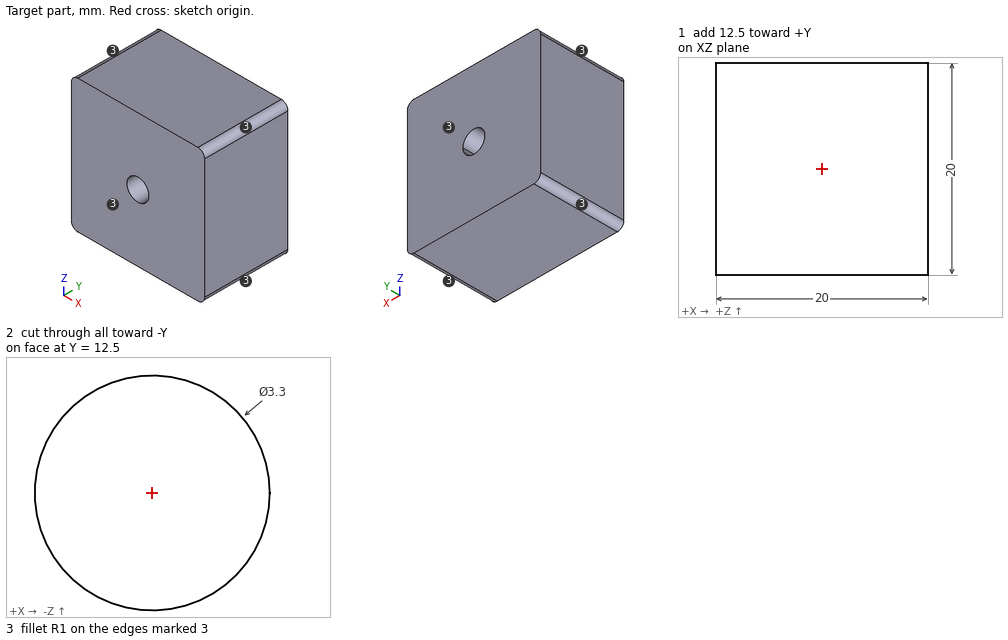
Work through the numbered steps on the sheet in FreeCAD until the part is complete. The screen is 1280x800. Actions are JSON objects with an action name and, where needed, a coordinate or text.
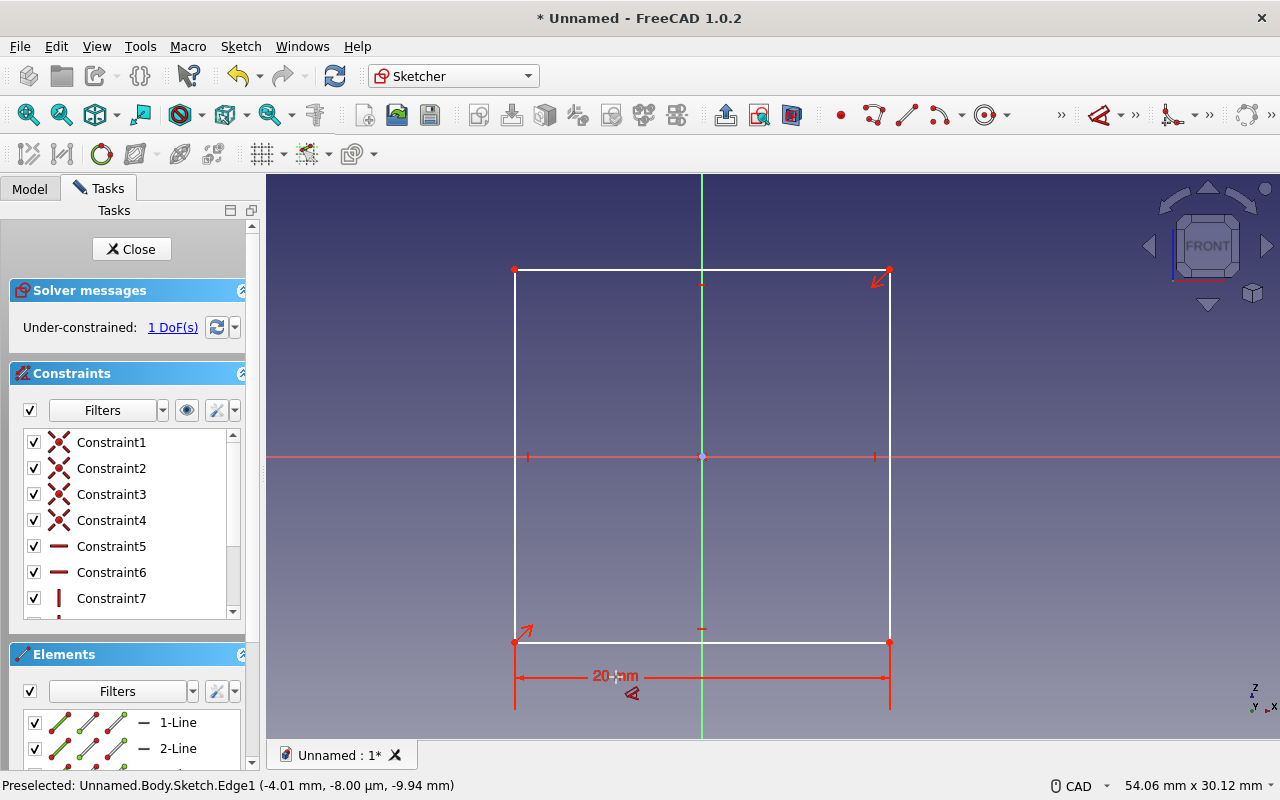
{"action": "left_click", "coordinate": [890, 531]}
{"action": "left_click", "coordinate": [924, 371]}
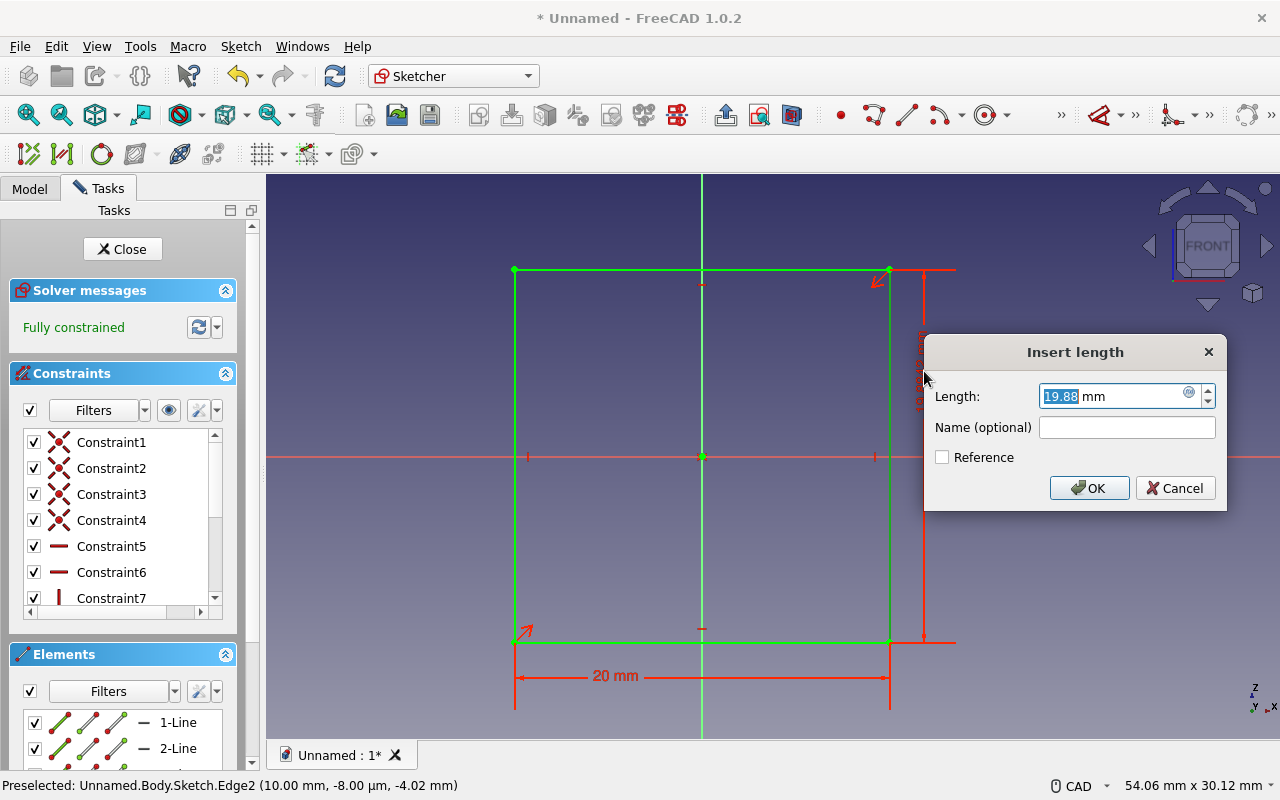
{"action": "type", "text": "20"}
{"action": "key", "text": "Return"}
{"action": "key", "text": "Escape"}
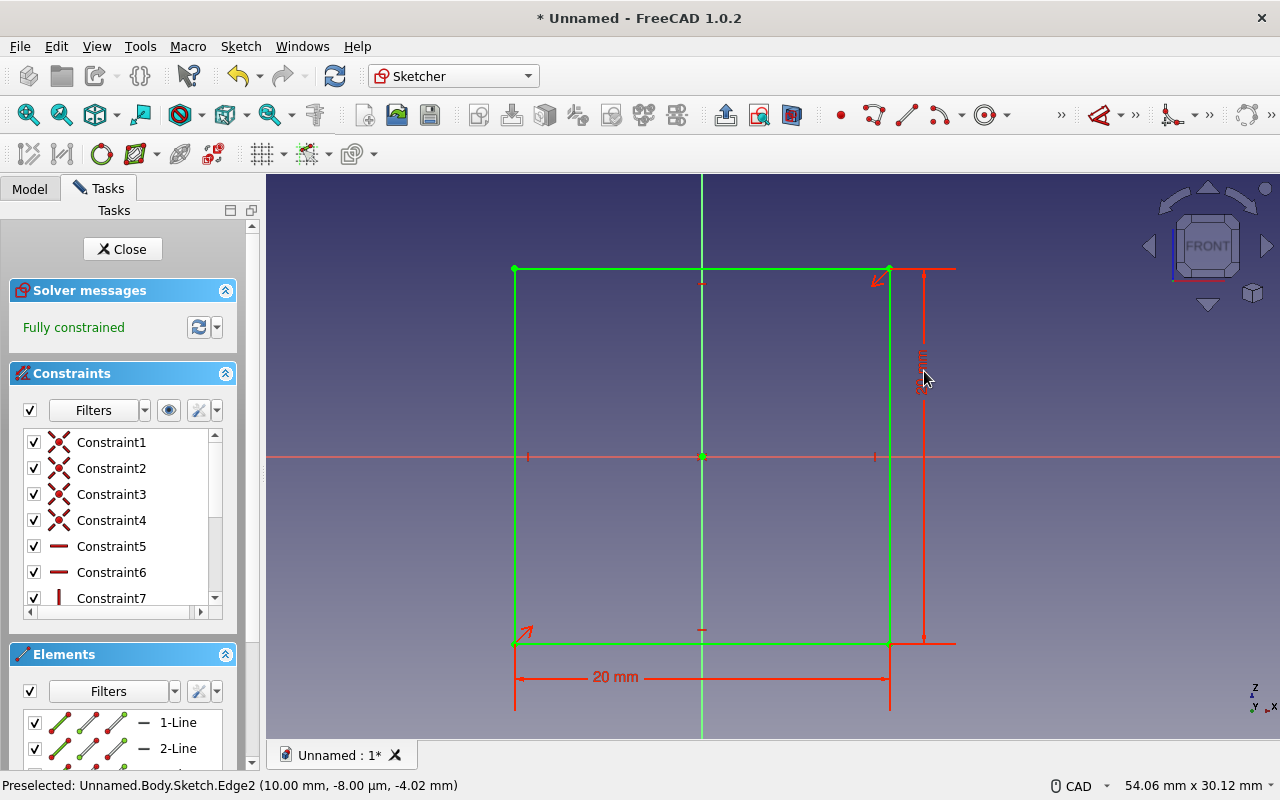
{"action": "left_click", "coordinate": [123, 249]}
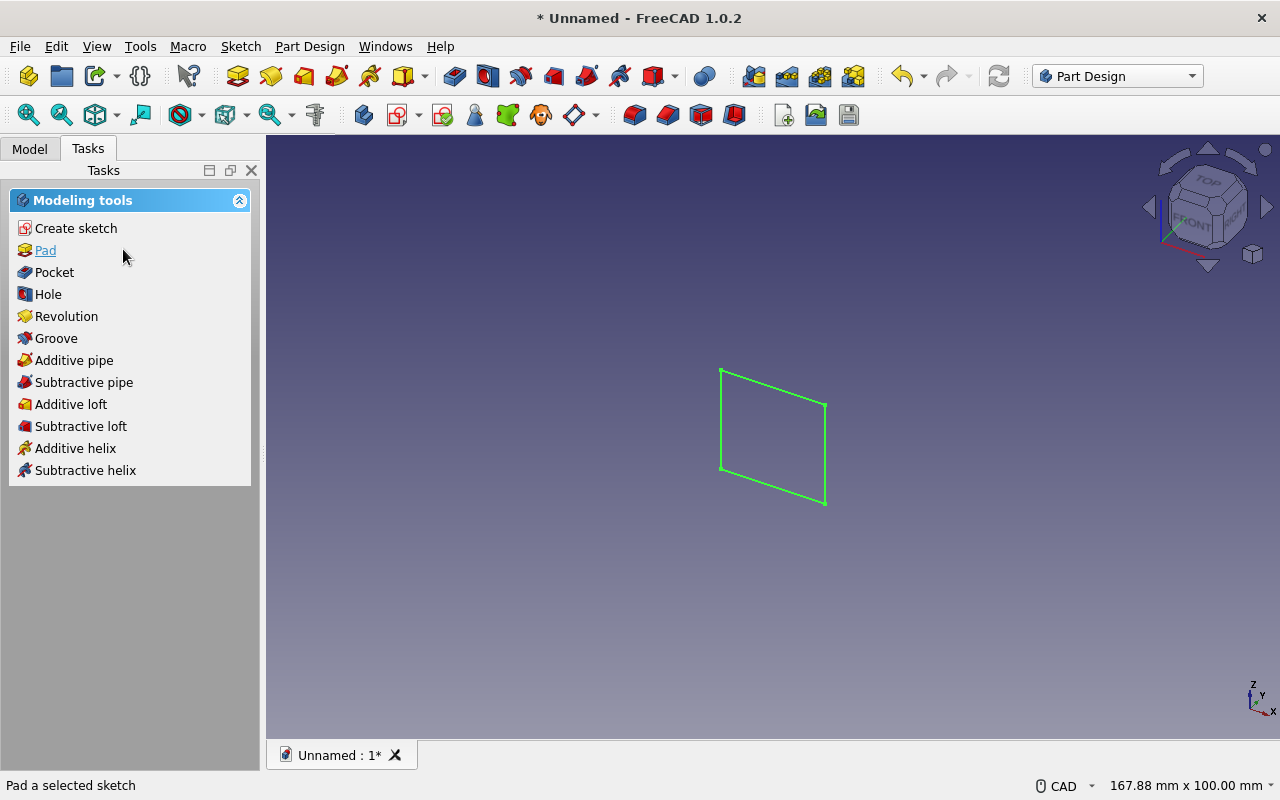
{"action": "left_click", "coordinate": [238, 76]}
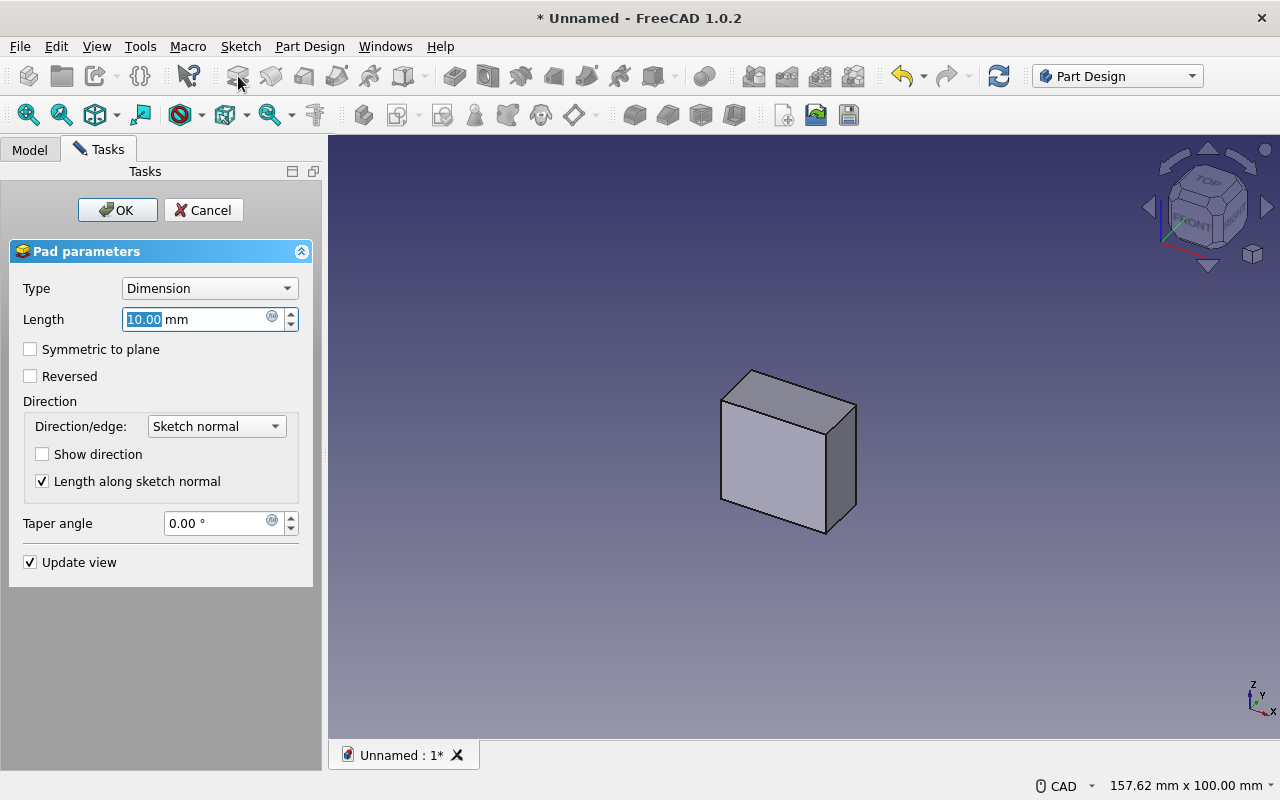
{"action": "type", "text": "12.5"}
{"action": "key", "text": "Tab"}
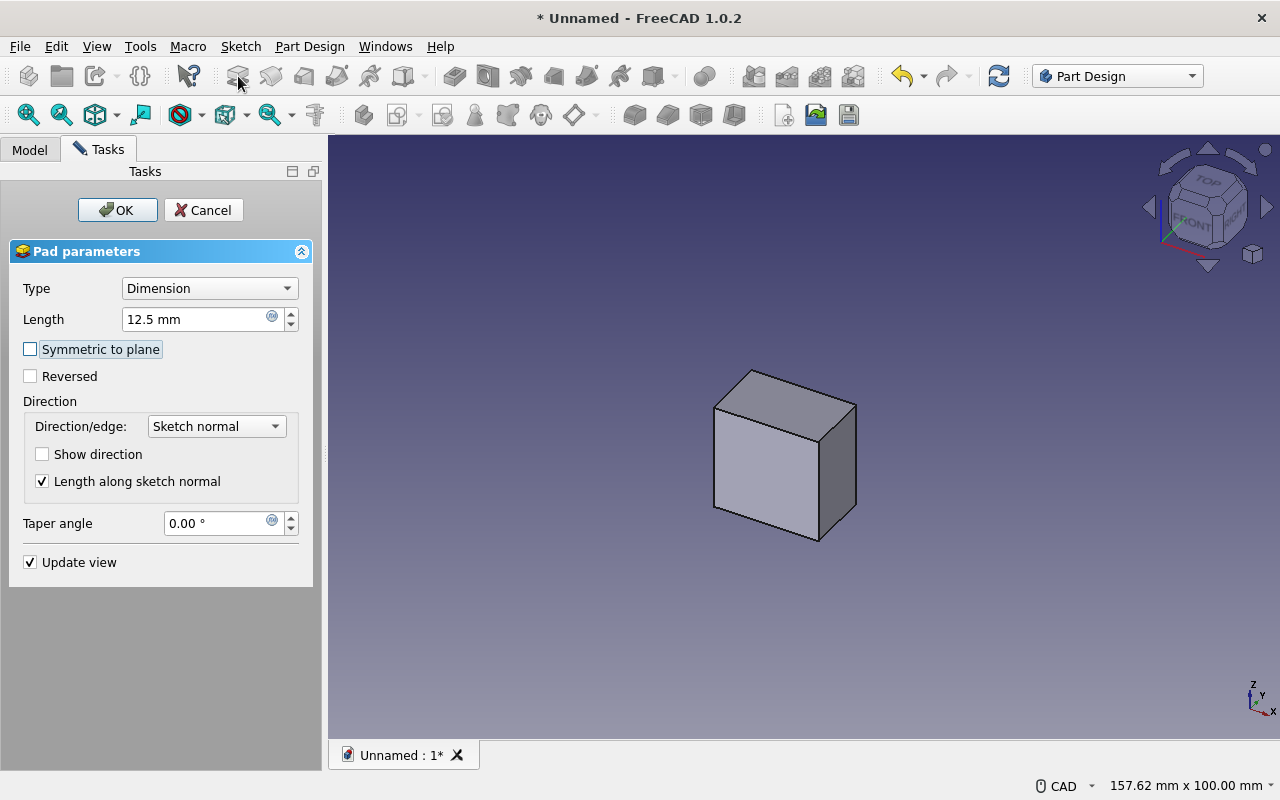
{"action": "left_click", "coordinate": [31, 376]}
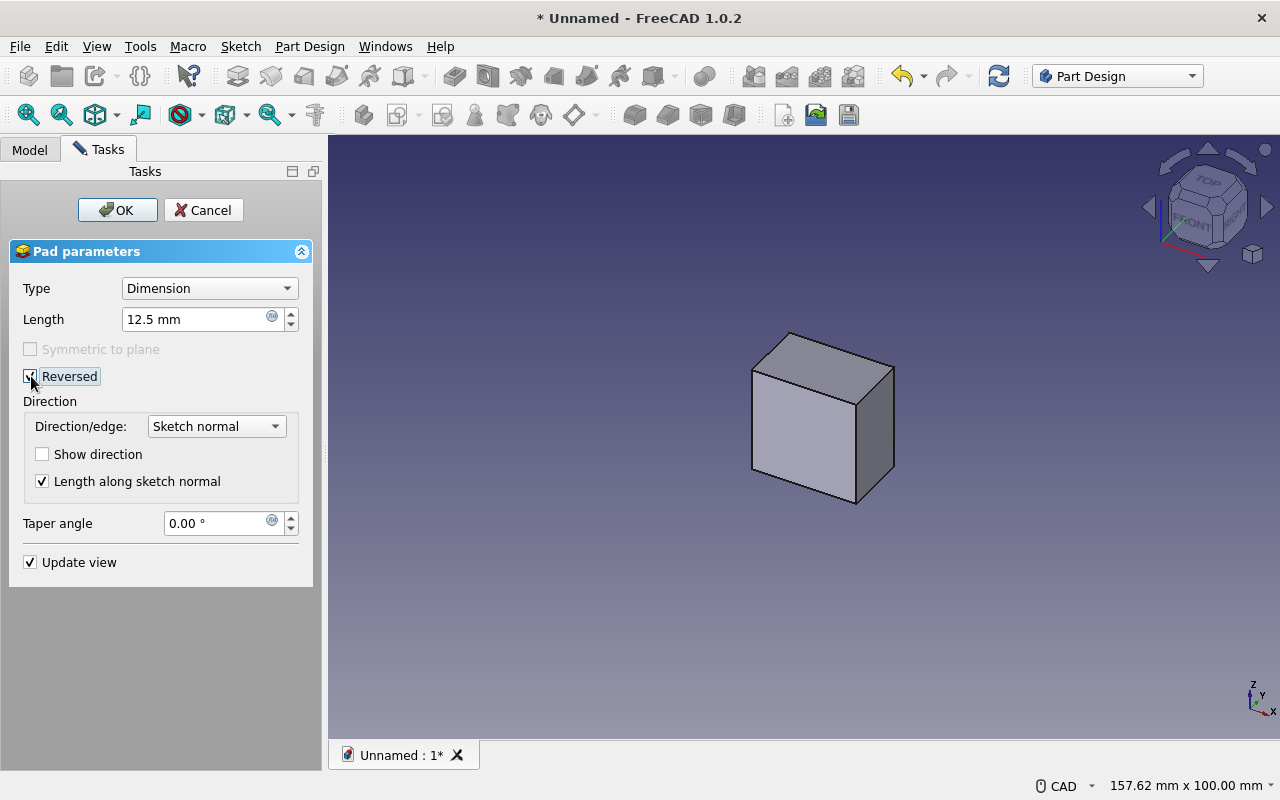
{"action": "left_click", "coordinate": [118, 210]}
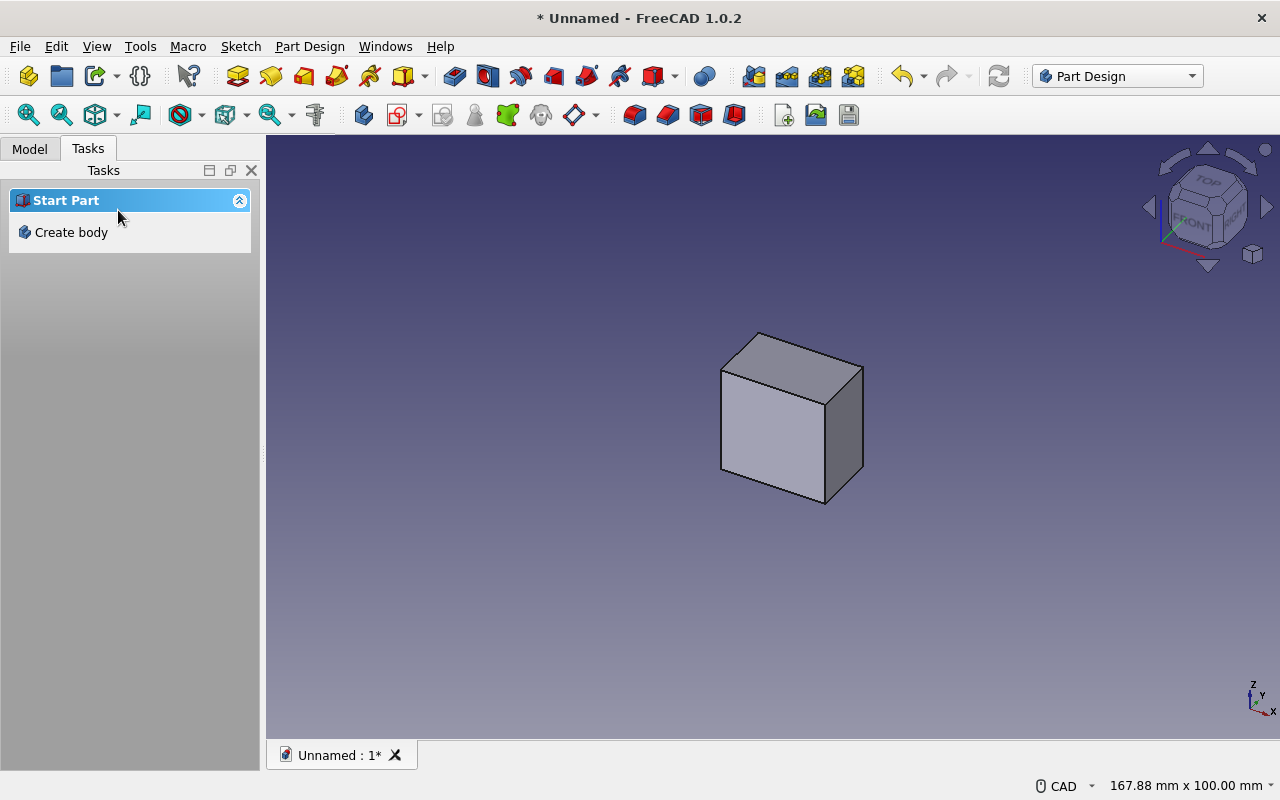
{"action": "left_click", "coordinate": [29, 116]}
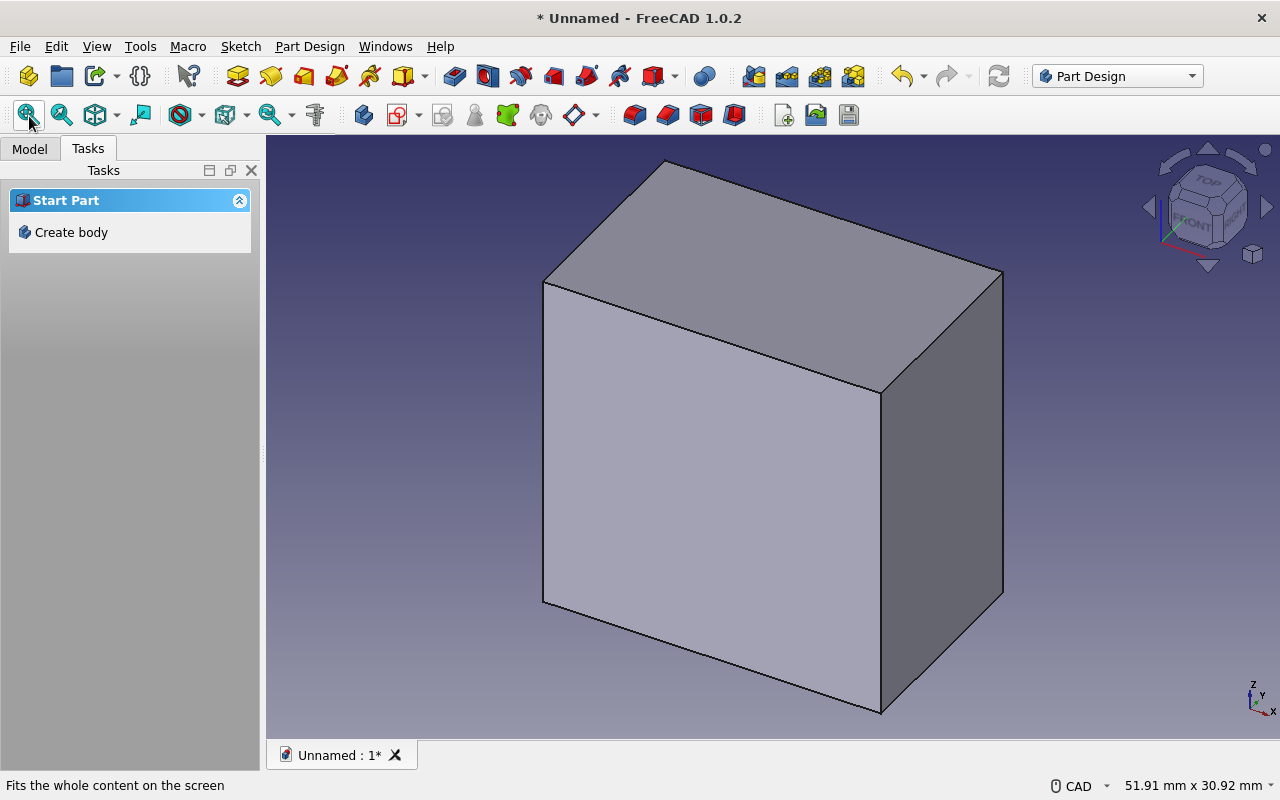
{"action": "key", "text": "4"}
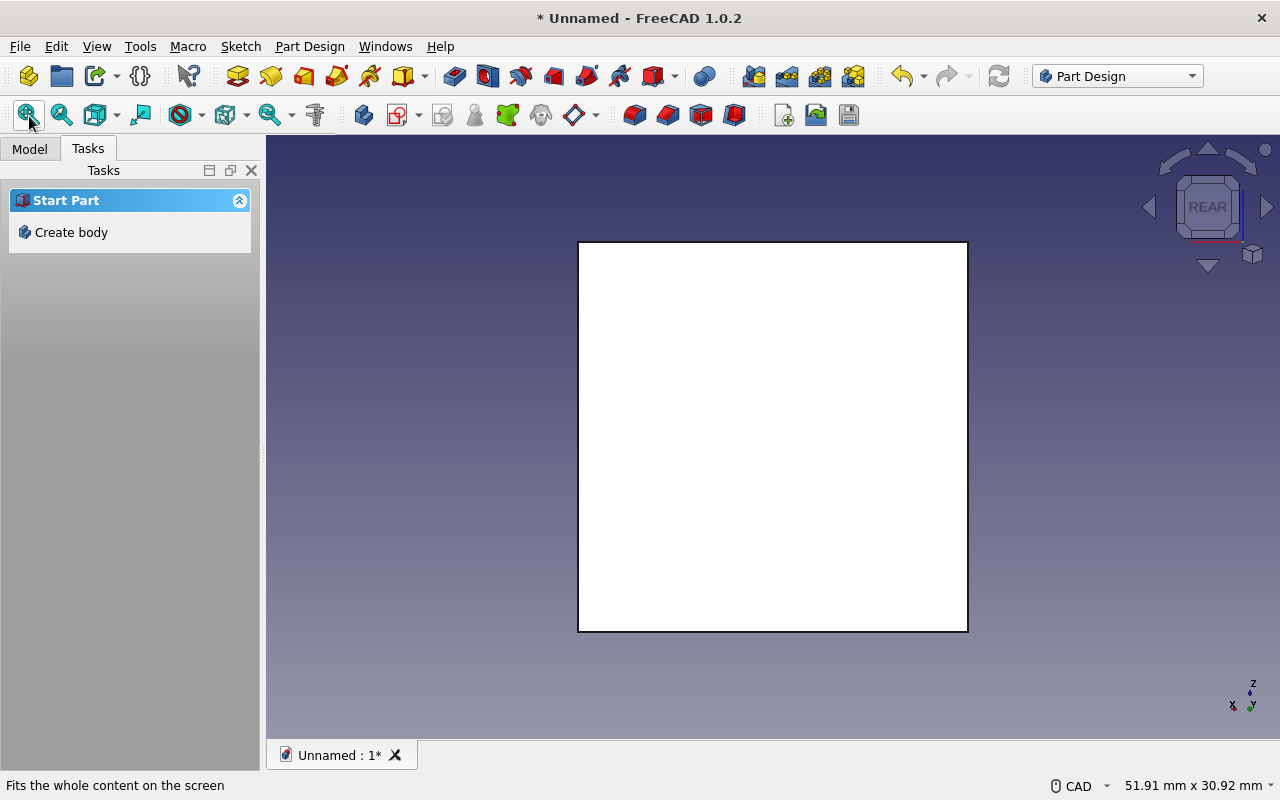
{"action": "left_click", "coordinate": [773, 436]}